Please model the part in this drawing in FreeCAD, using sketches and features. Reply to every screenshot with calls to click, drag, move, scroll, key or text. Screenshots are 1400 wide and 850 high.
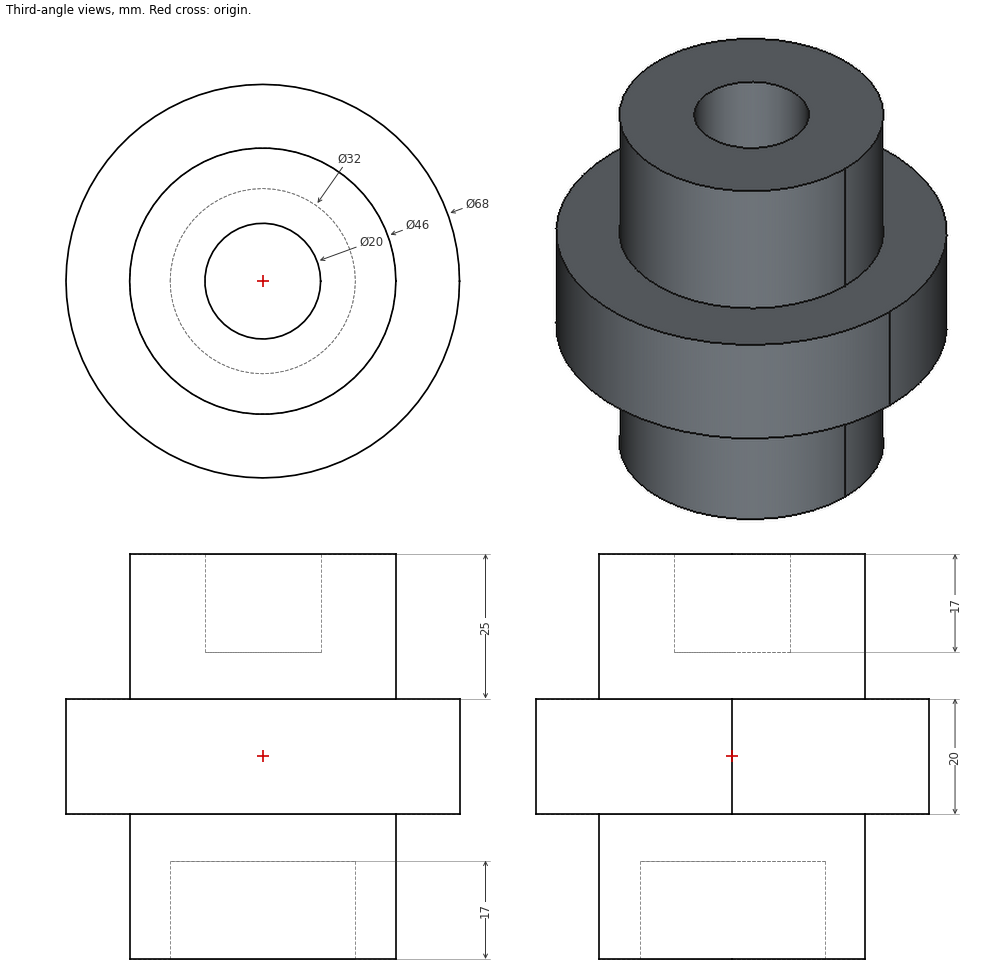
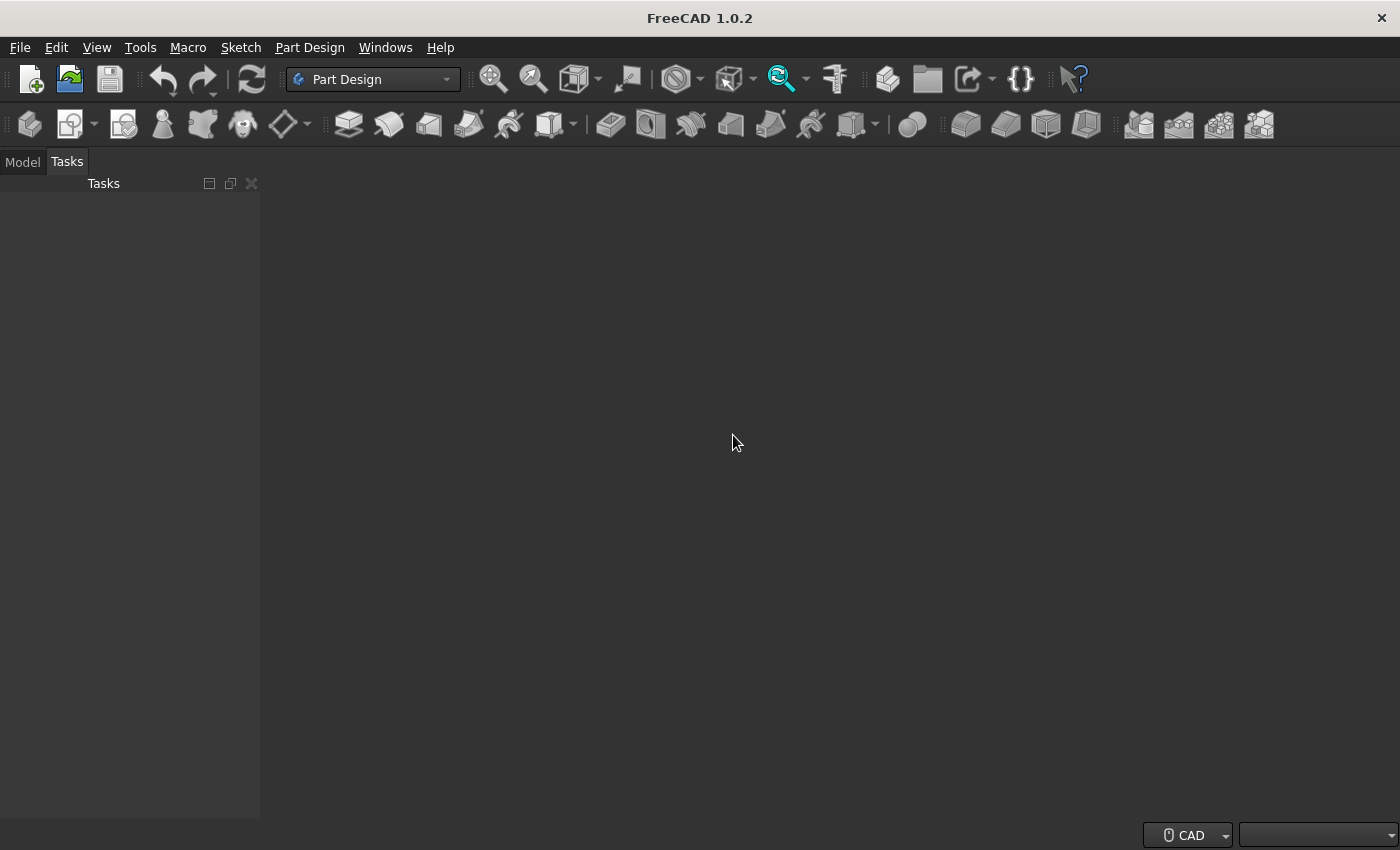
click(30, 80)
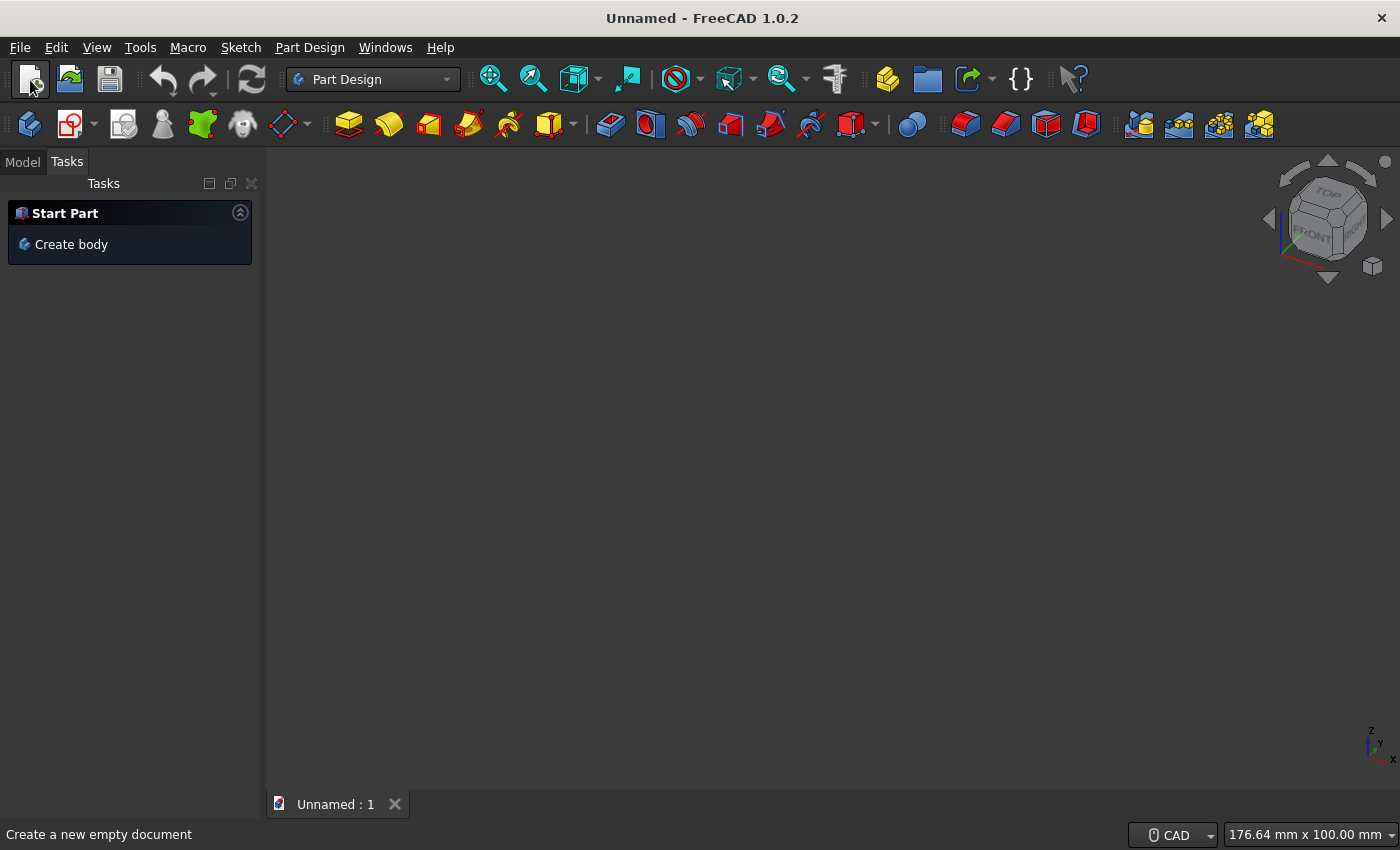
click(70, 124)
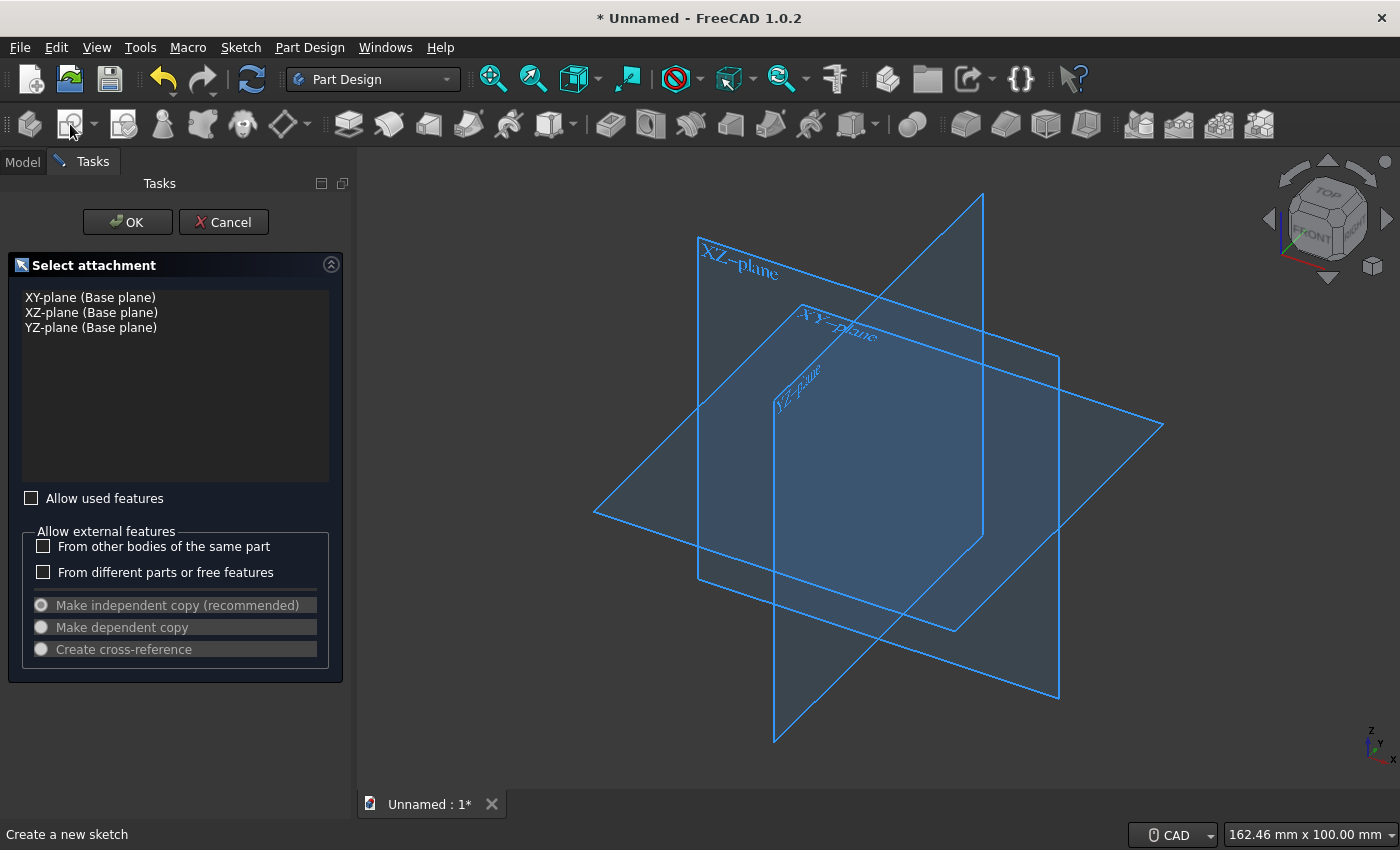
click(82, 298)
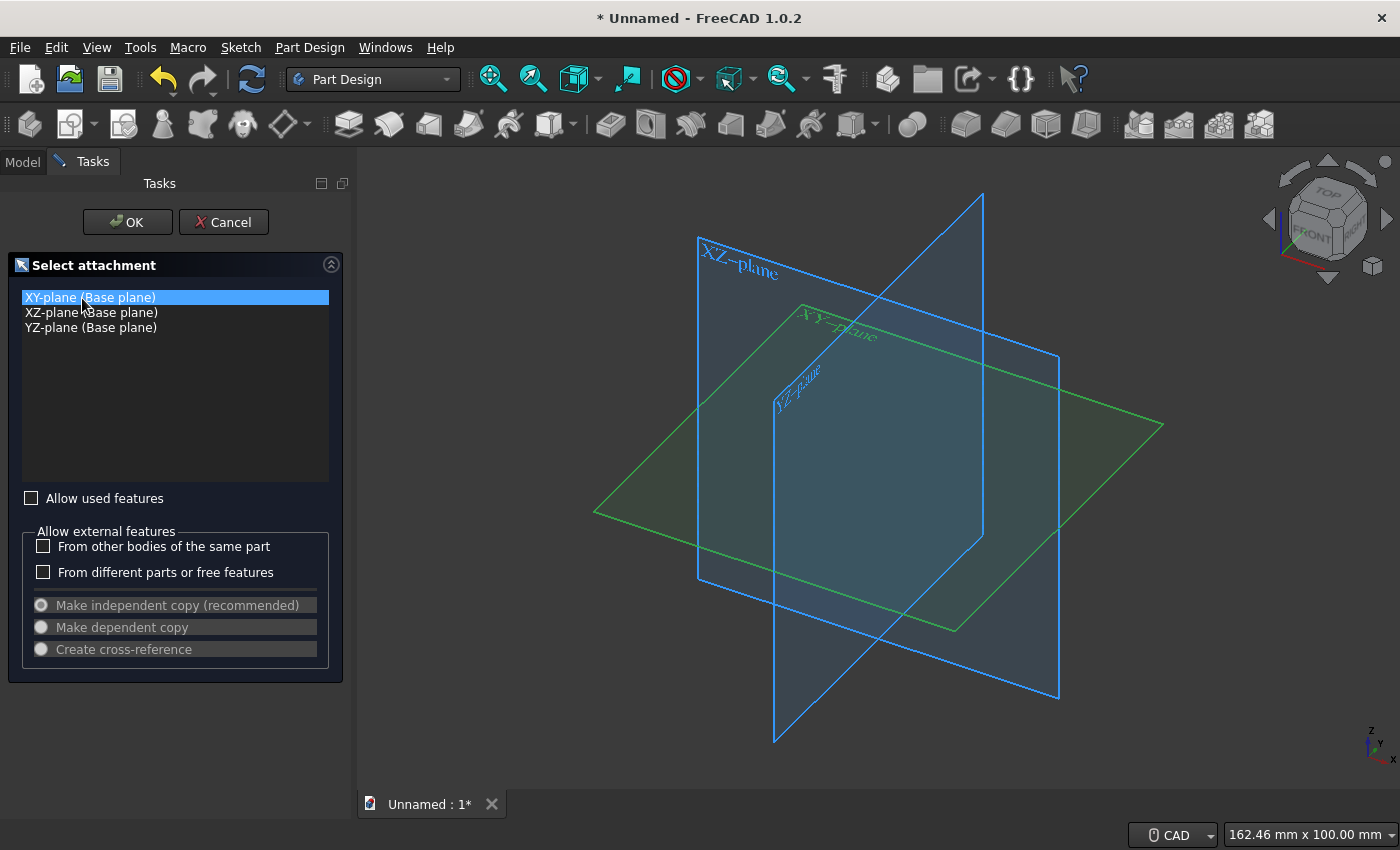
click(128, 222)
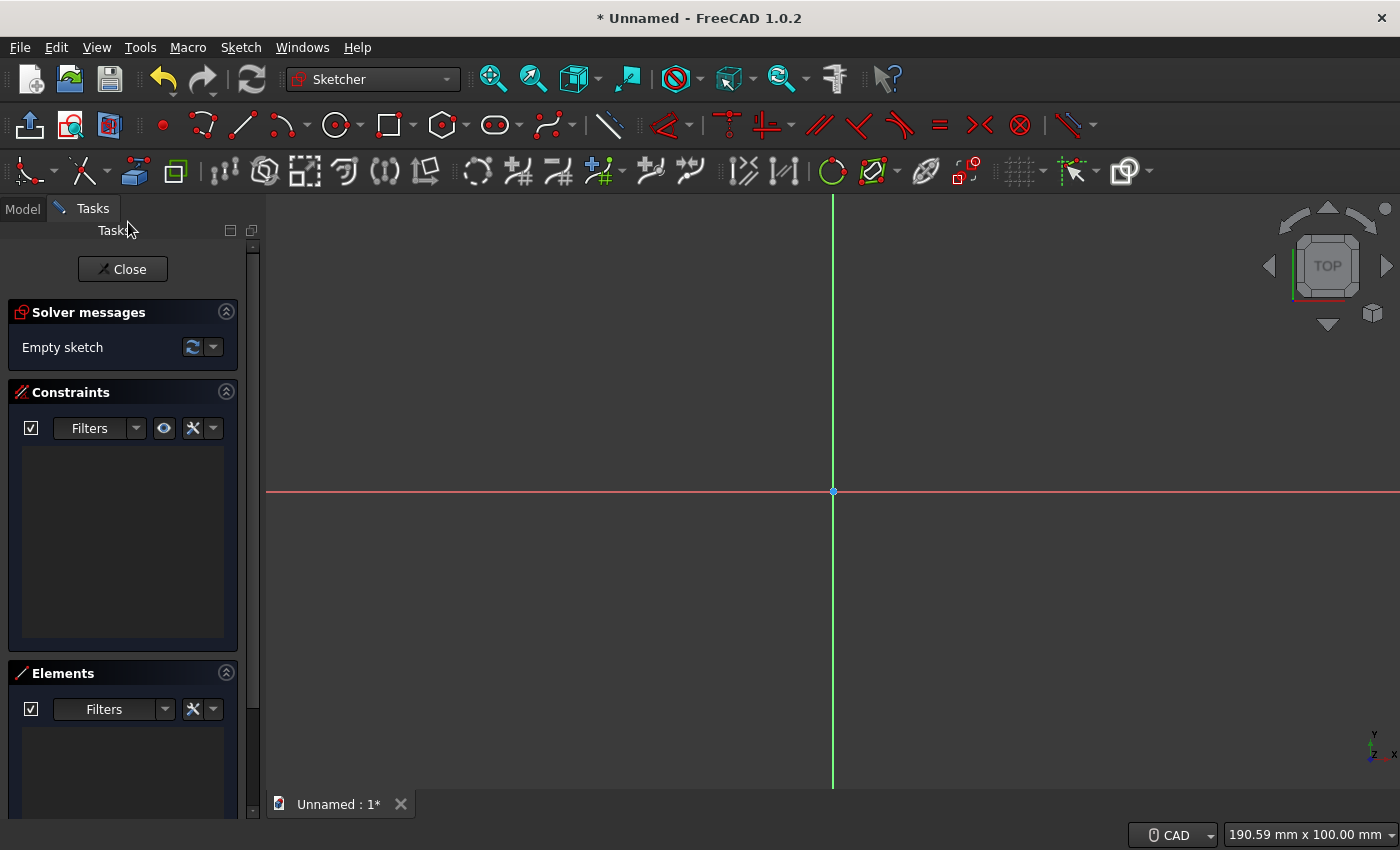
click(336, 126)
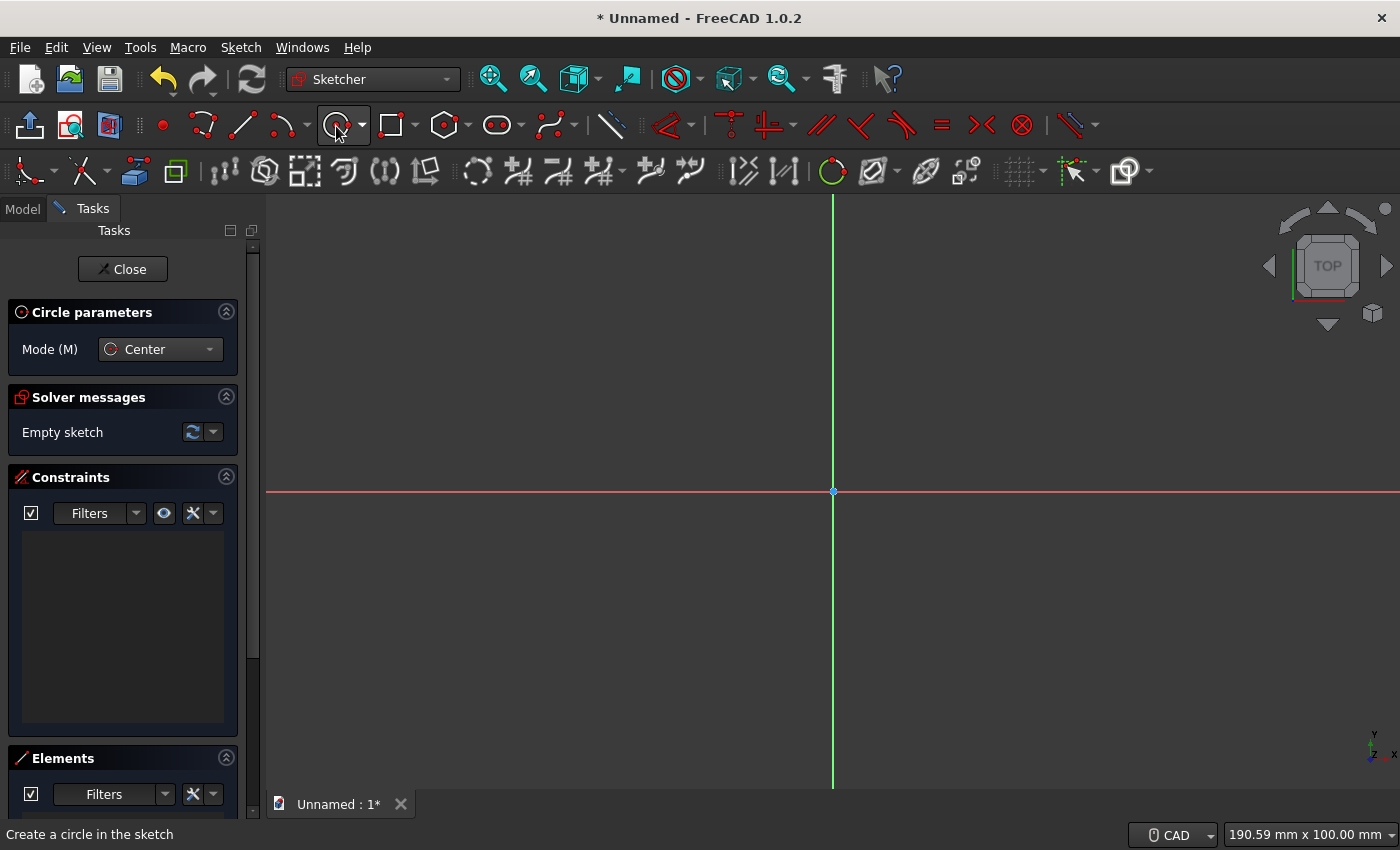
click(833, 492)
move(976, 348)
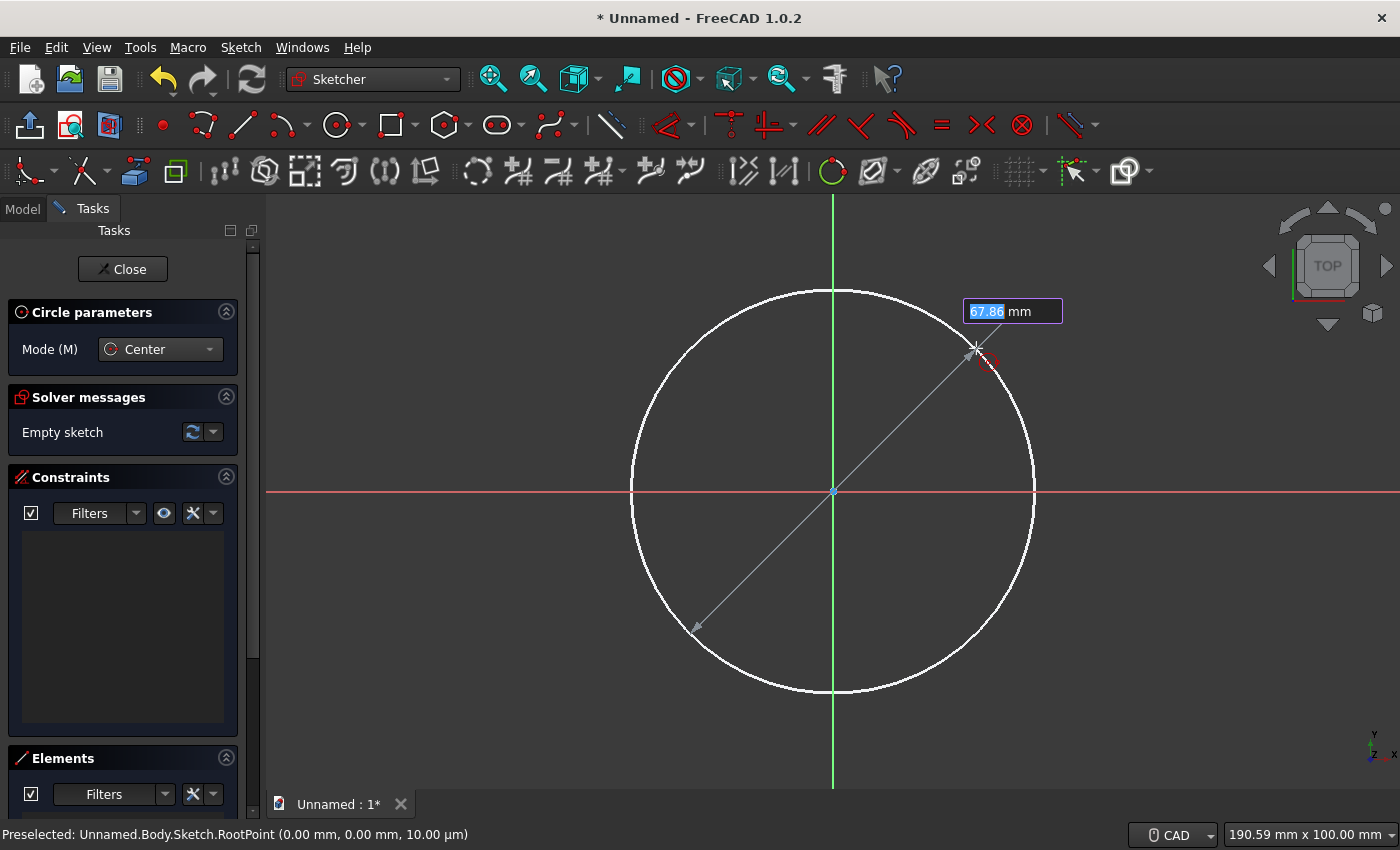
text(68)
key(Return)
key(Escape)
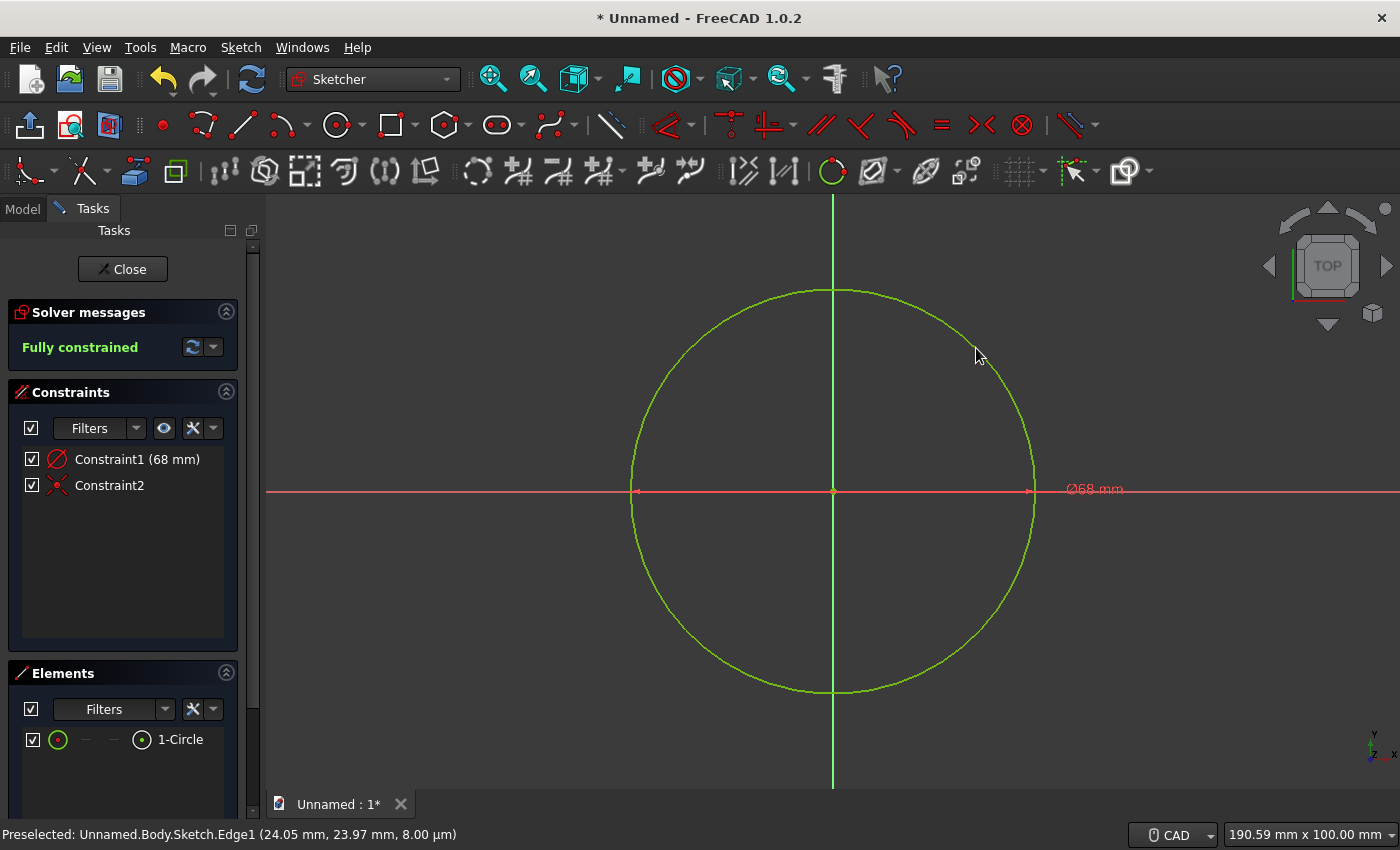
click(123, 269)